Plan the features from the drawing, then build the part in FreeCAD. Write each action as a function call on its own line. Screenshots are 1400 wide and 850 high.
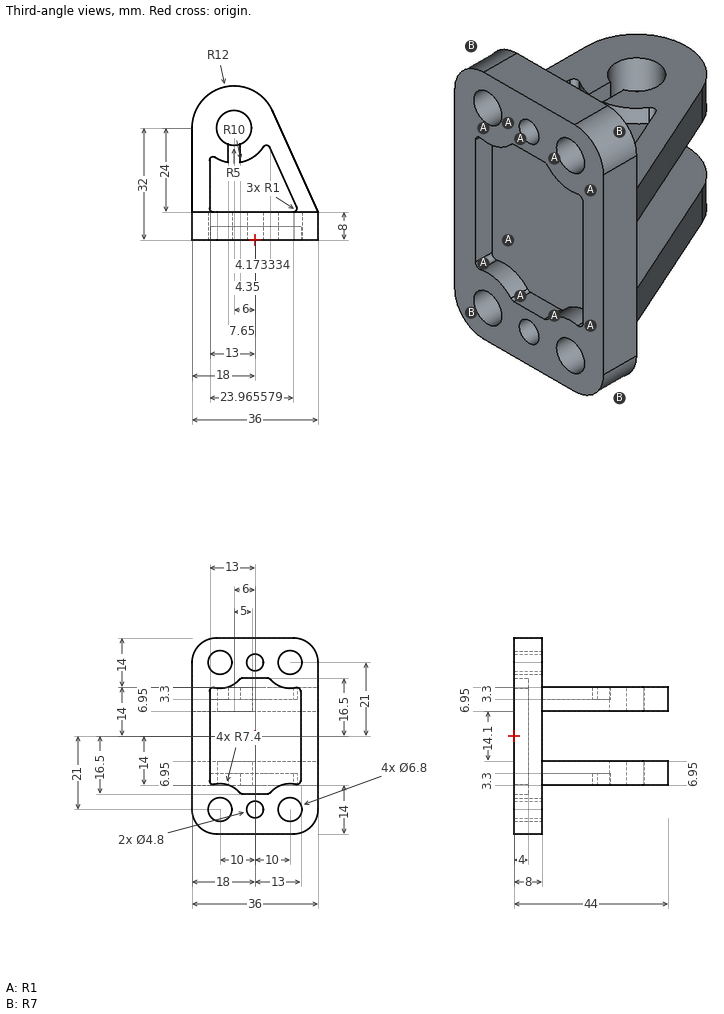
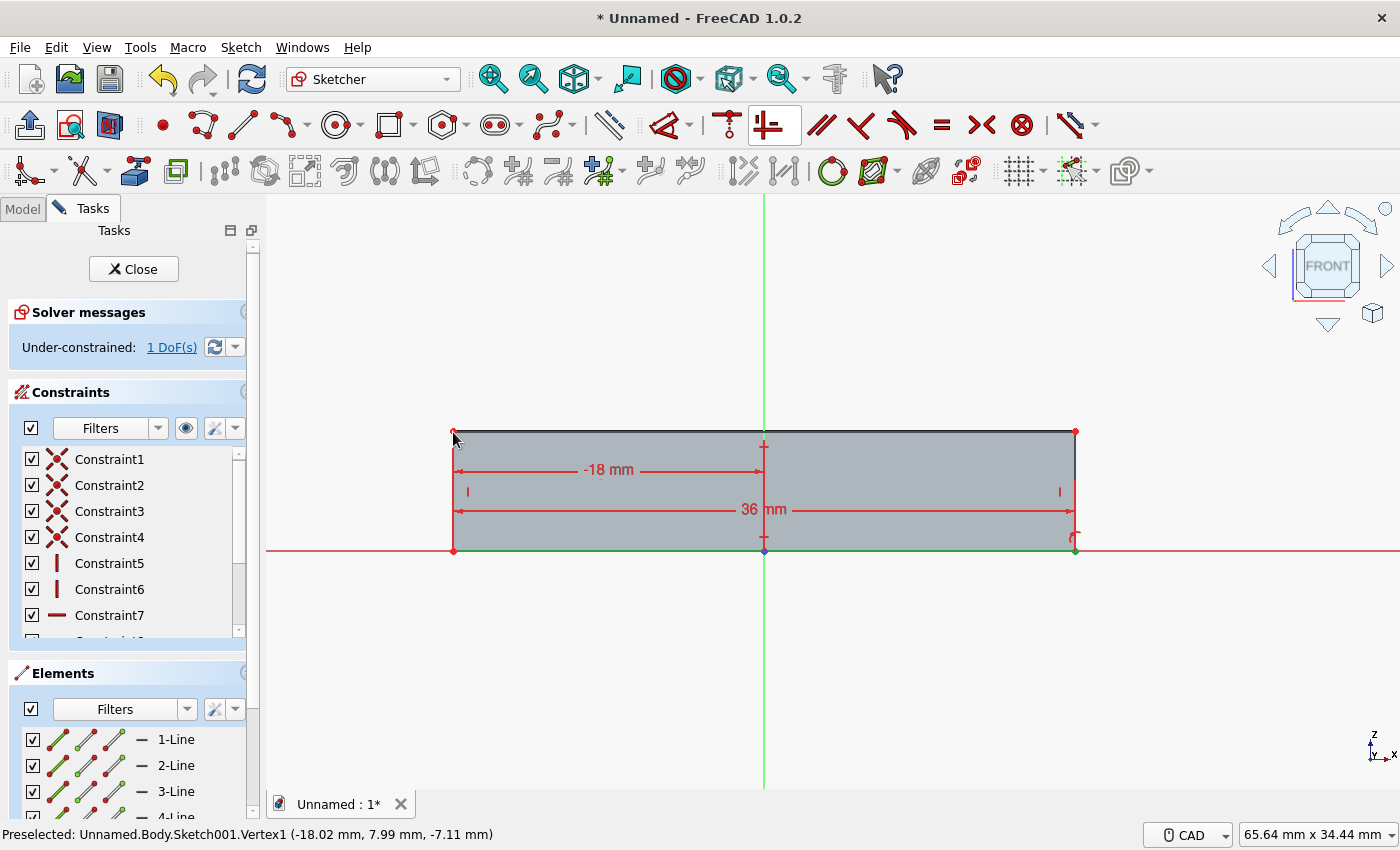
click(453, 468)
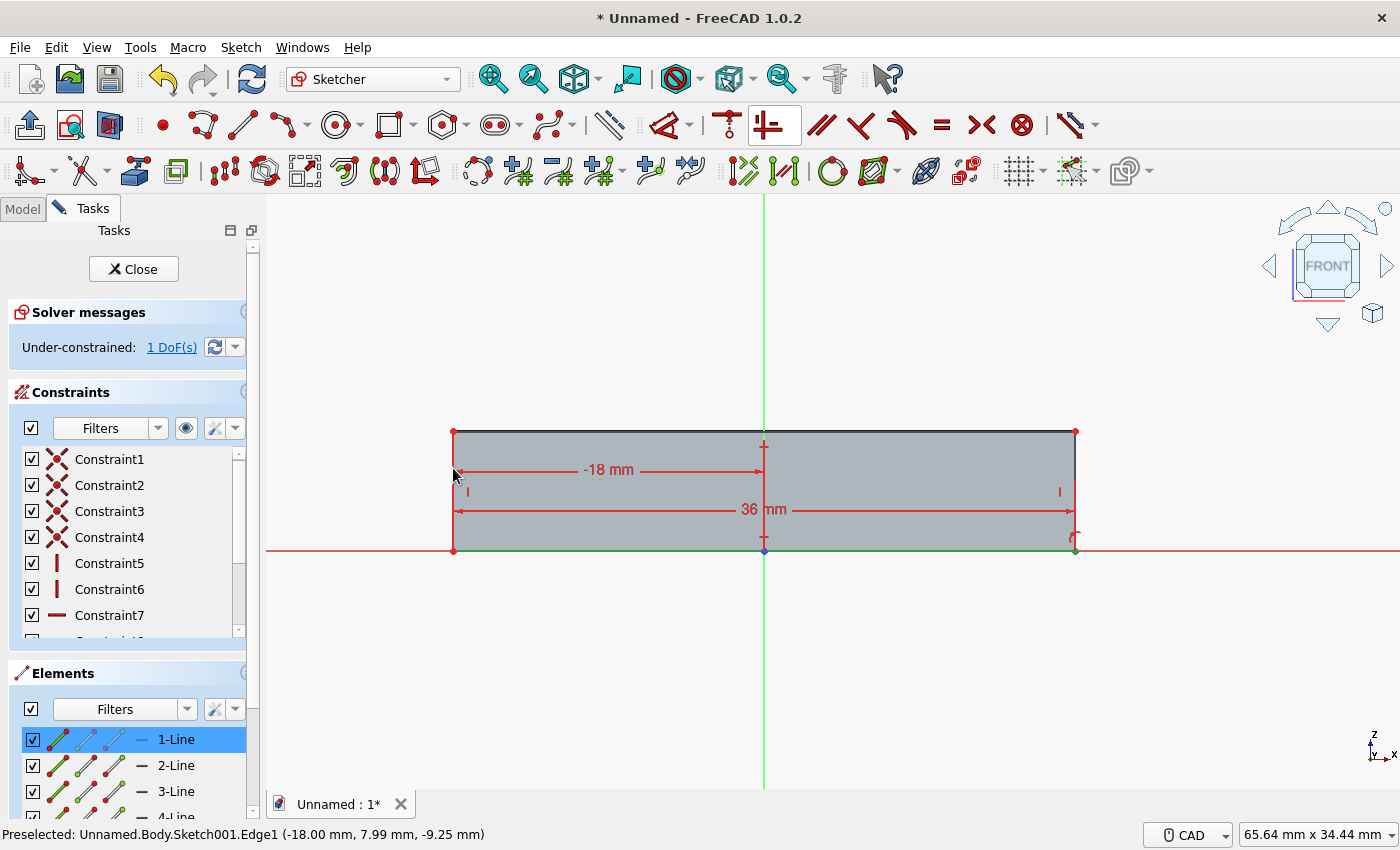
key(i)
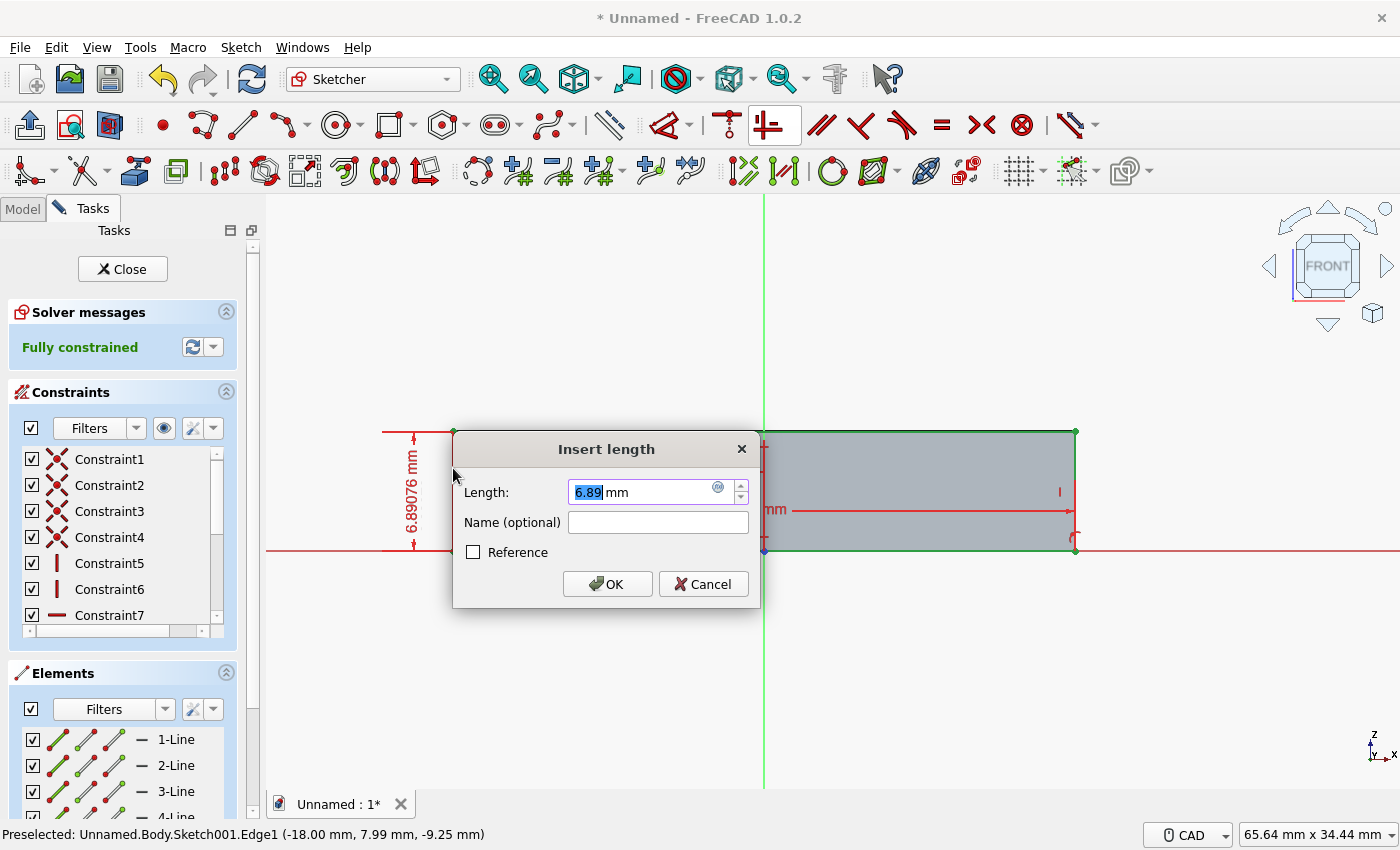
text(6.95)
key(Return)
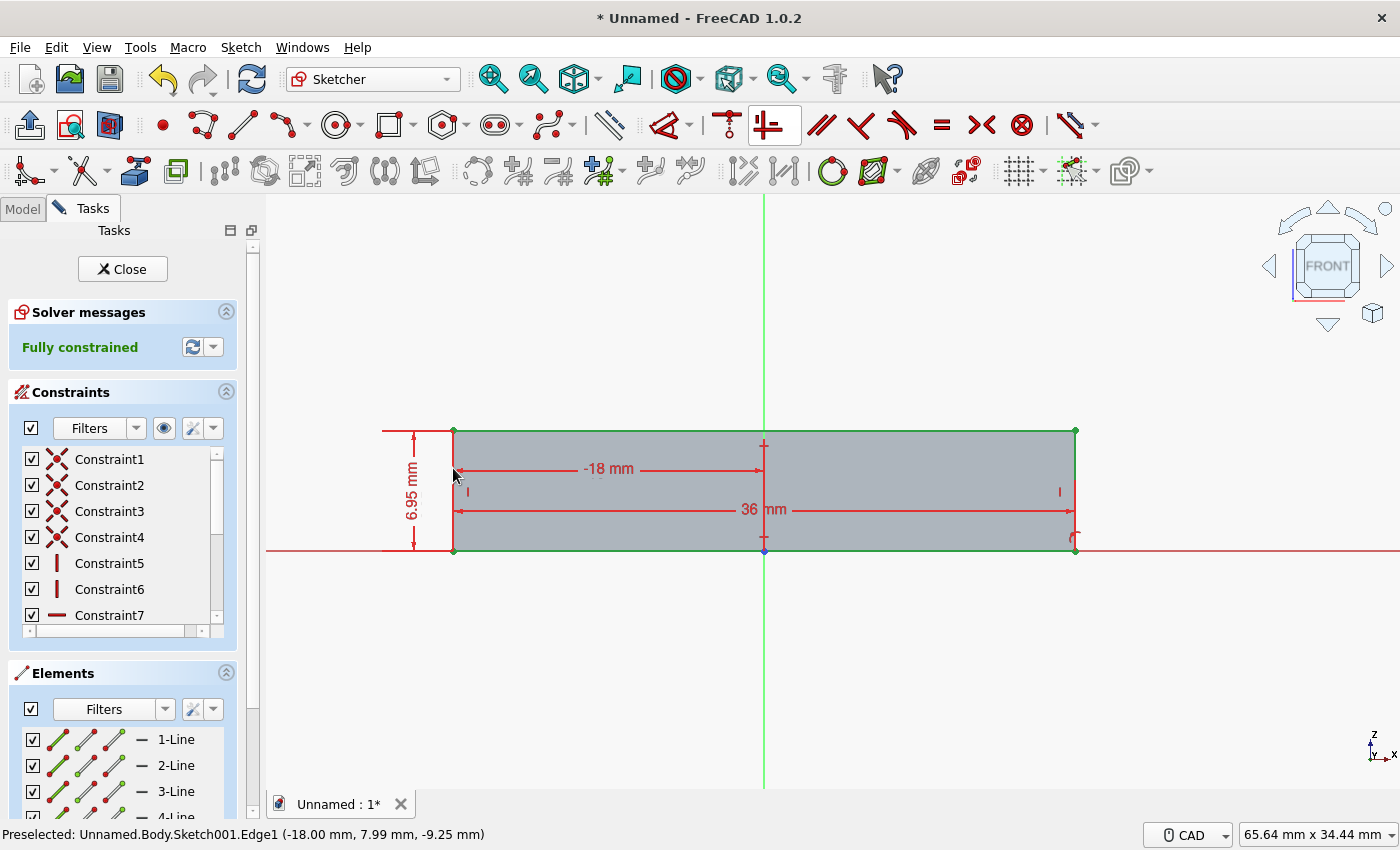
click(123, 269)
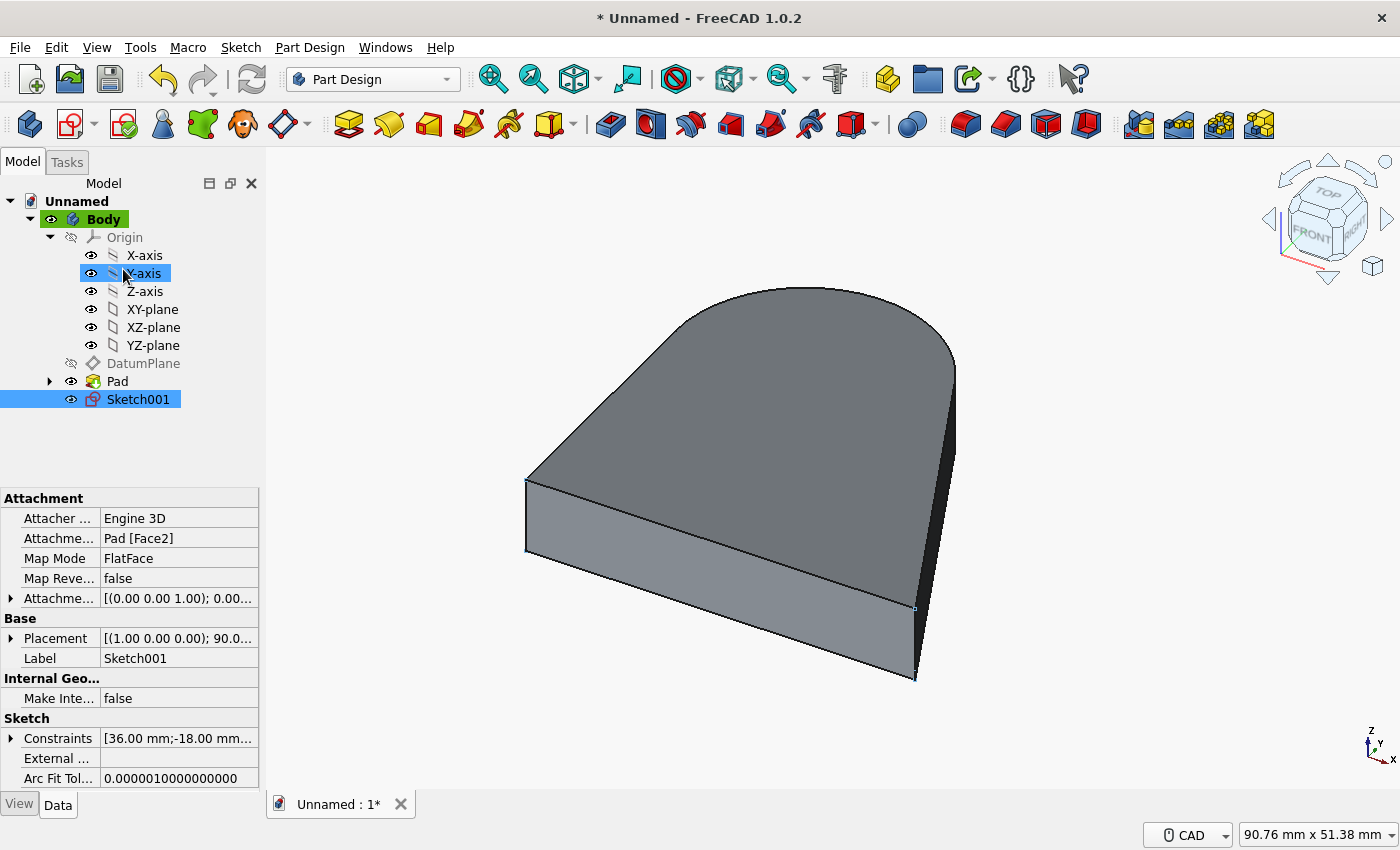
click(350, 124)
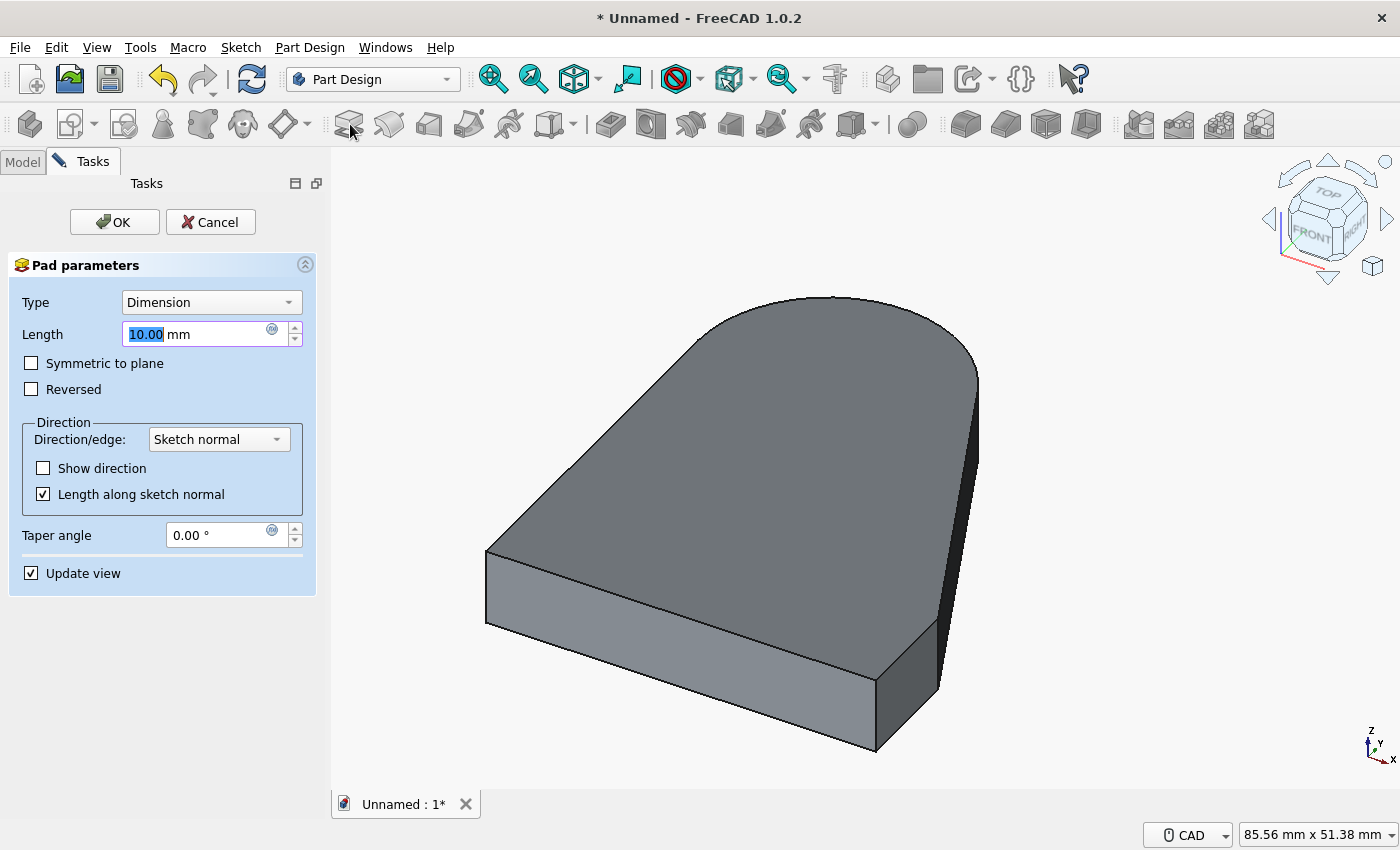
text(8)
key(Tab)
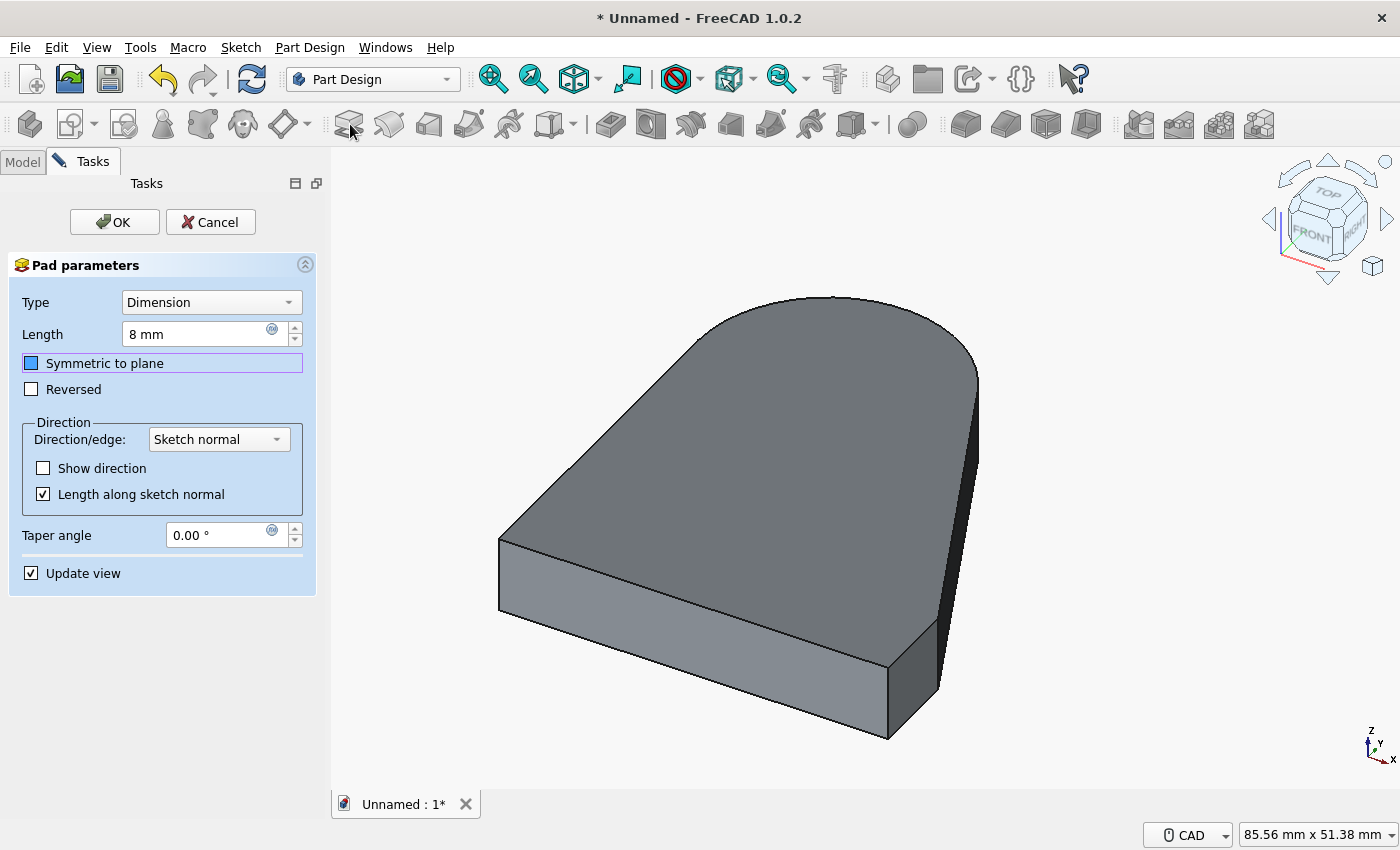
click(115, 222)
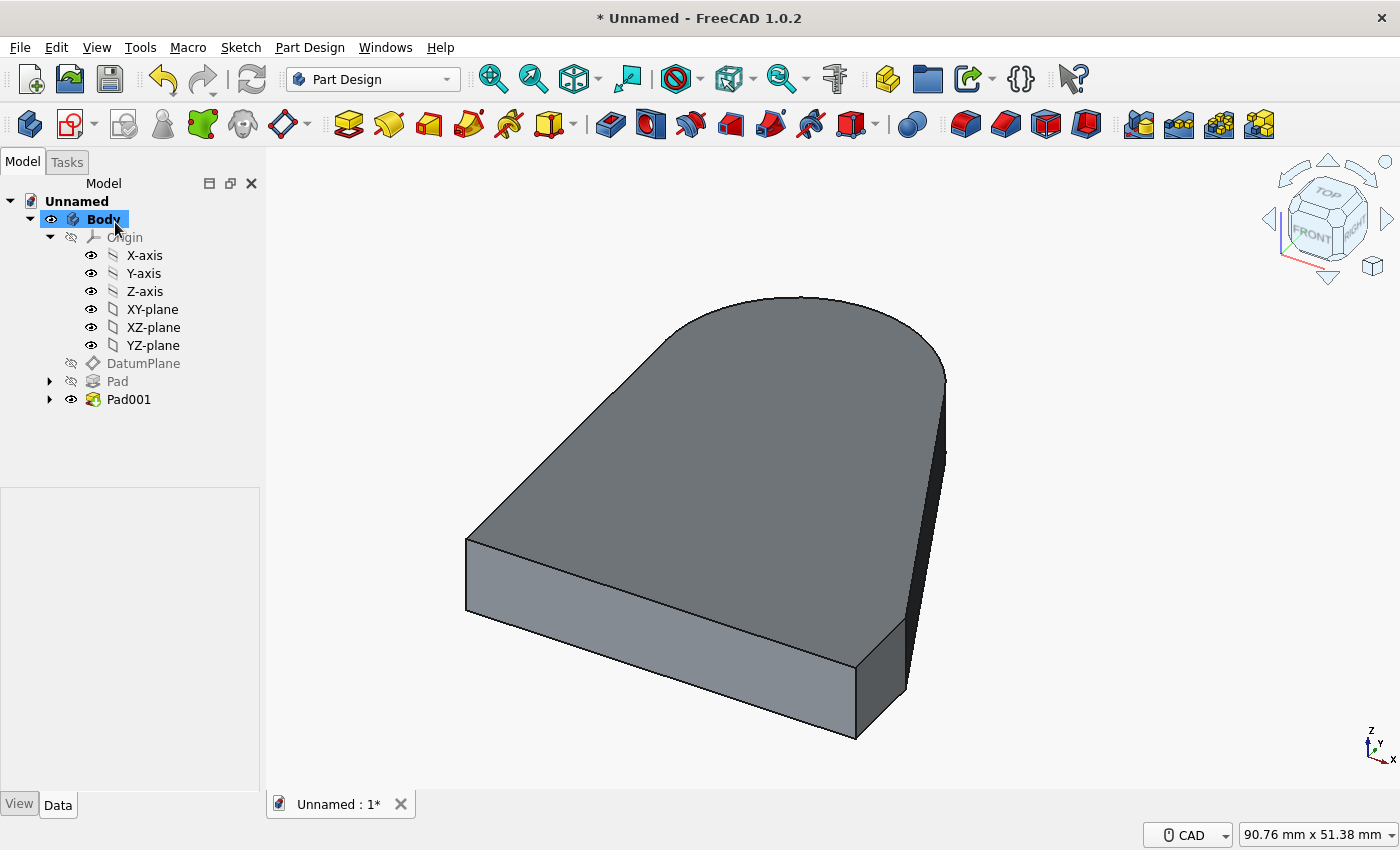
click(759, 505)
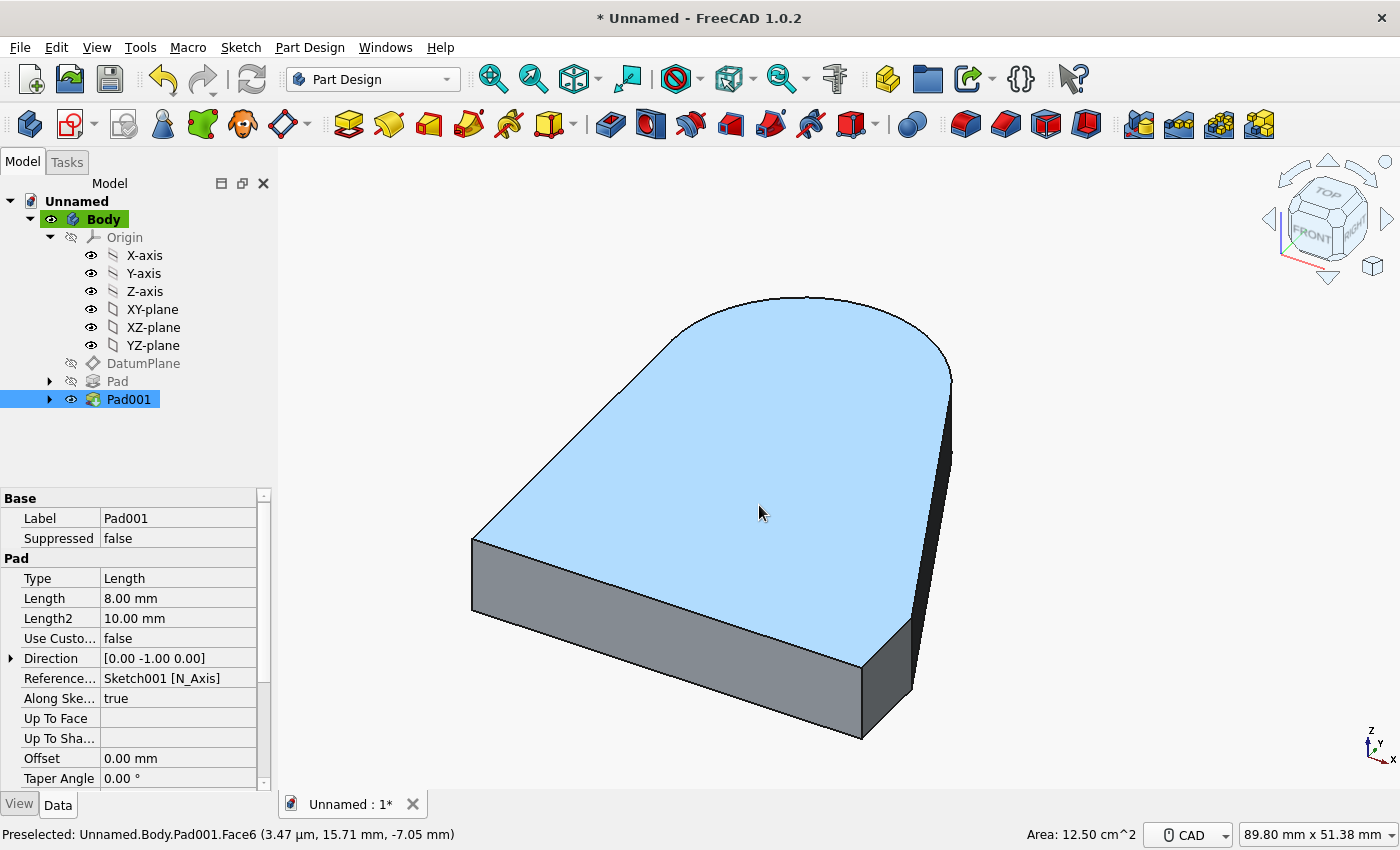
click(70, 124)